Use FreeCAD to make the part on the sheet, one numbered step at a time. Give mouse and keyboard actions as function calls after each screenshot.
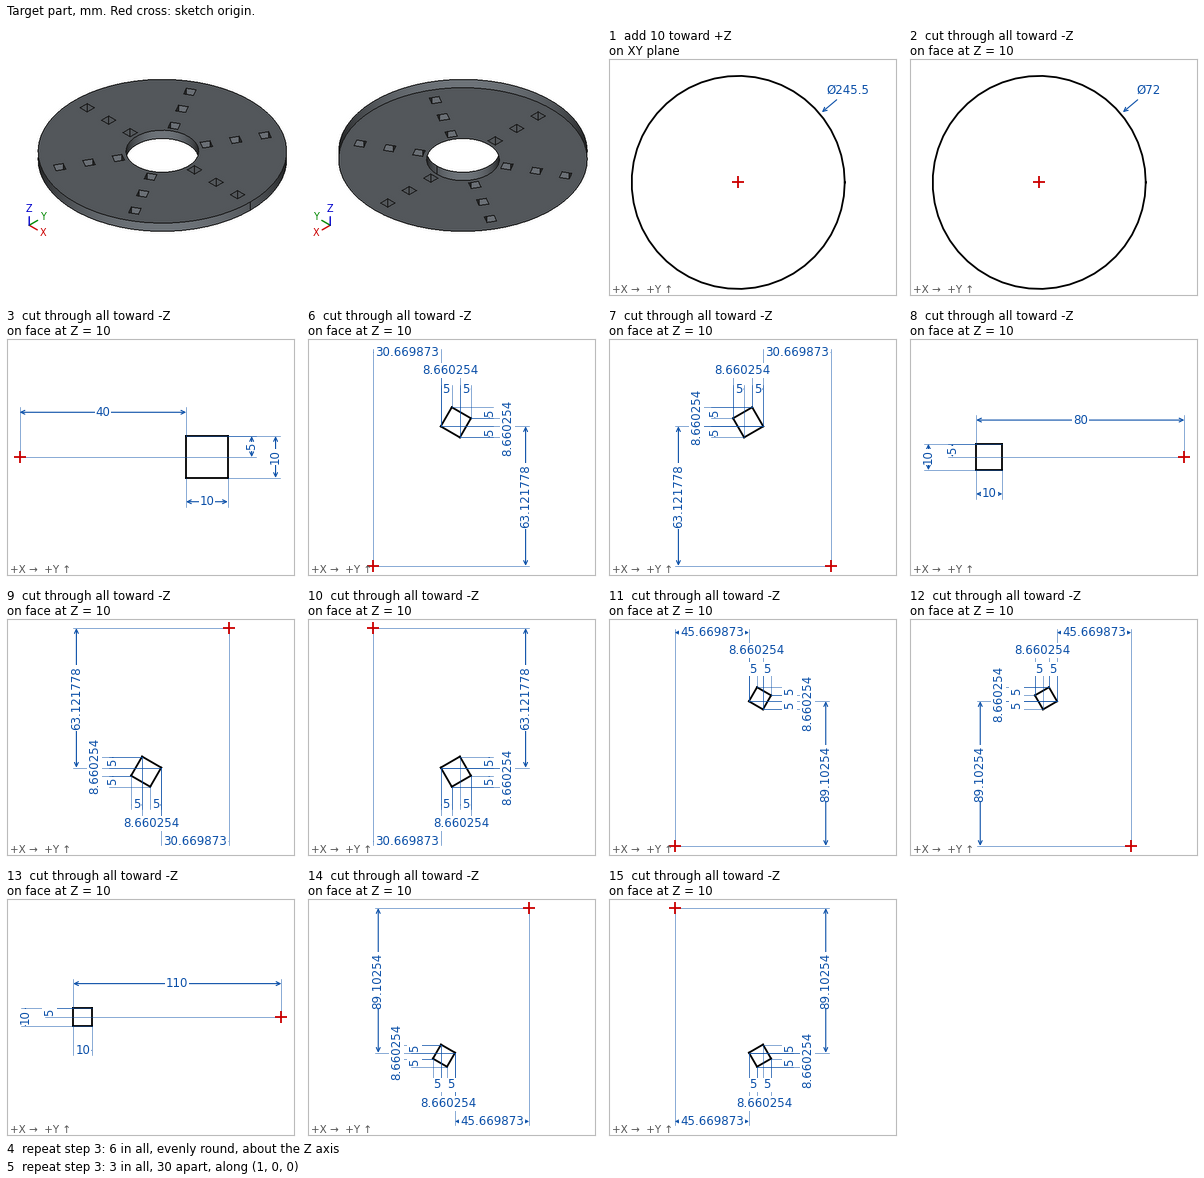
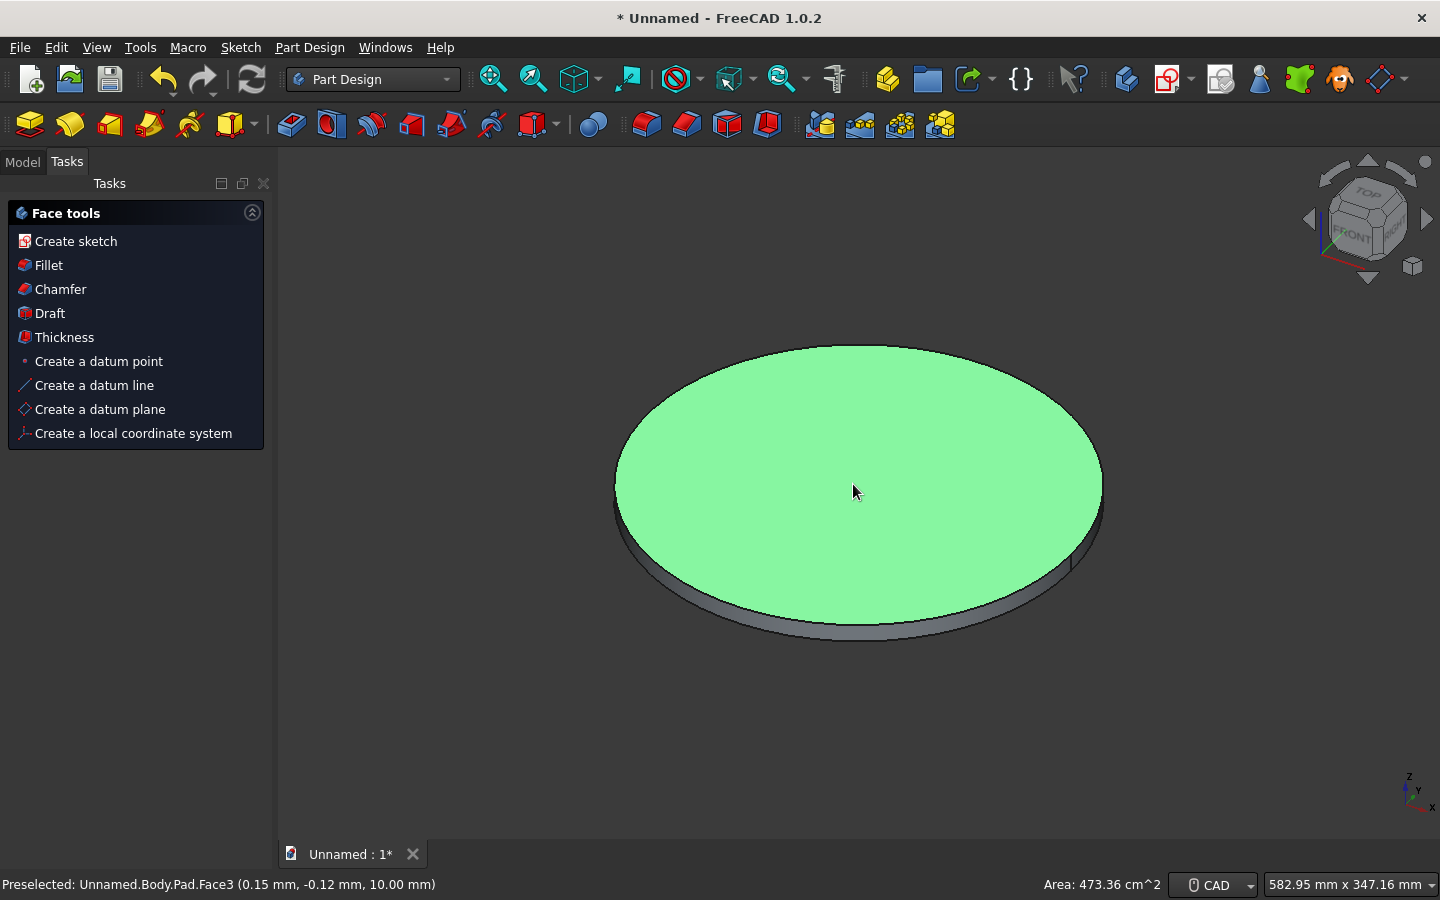
click(1168, 80)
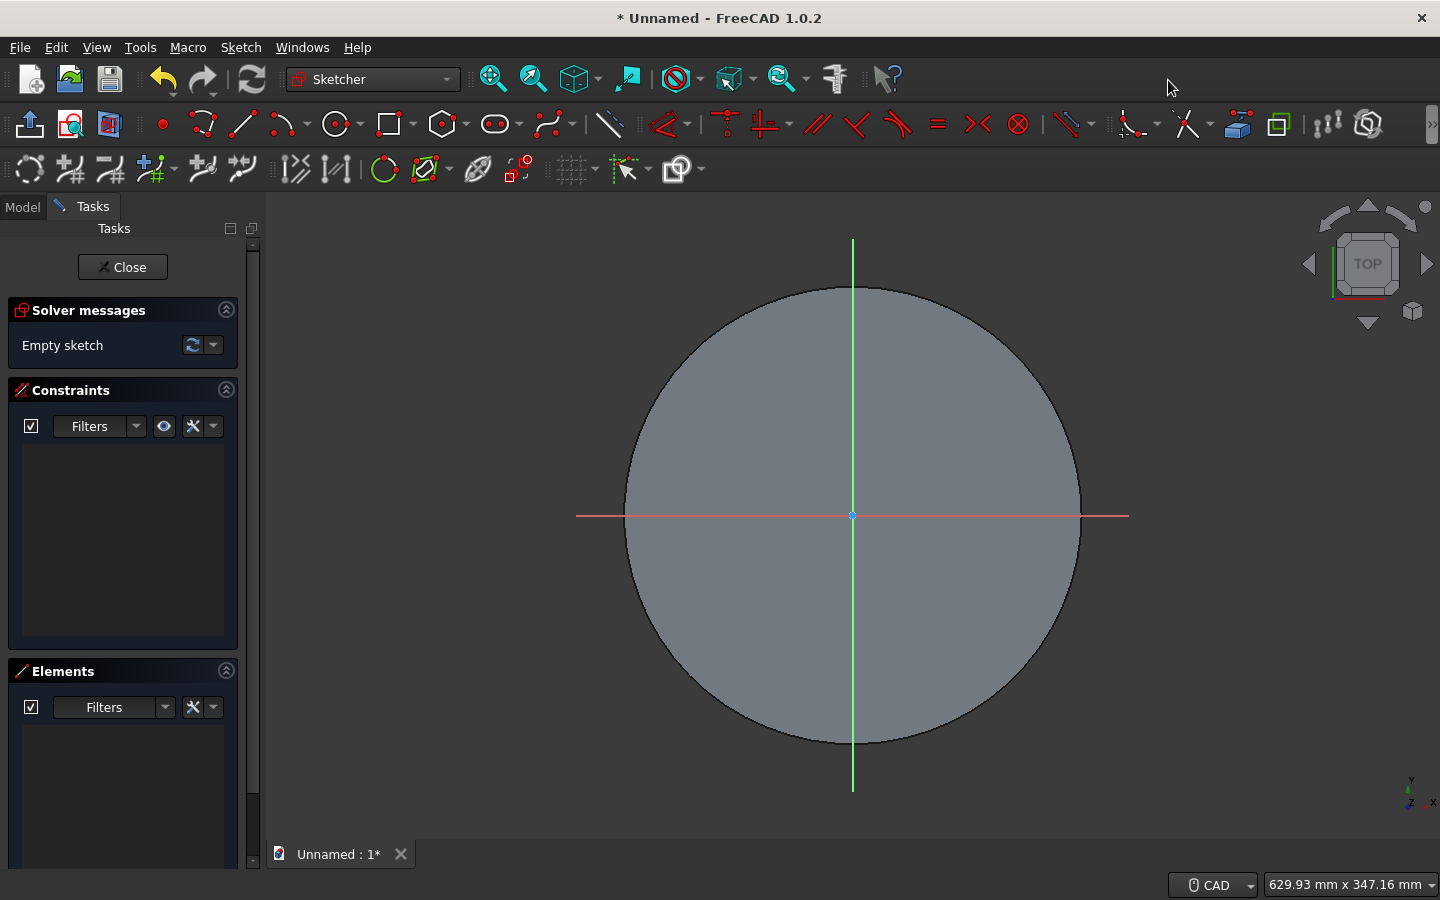
scroll(882, 516, up, 6)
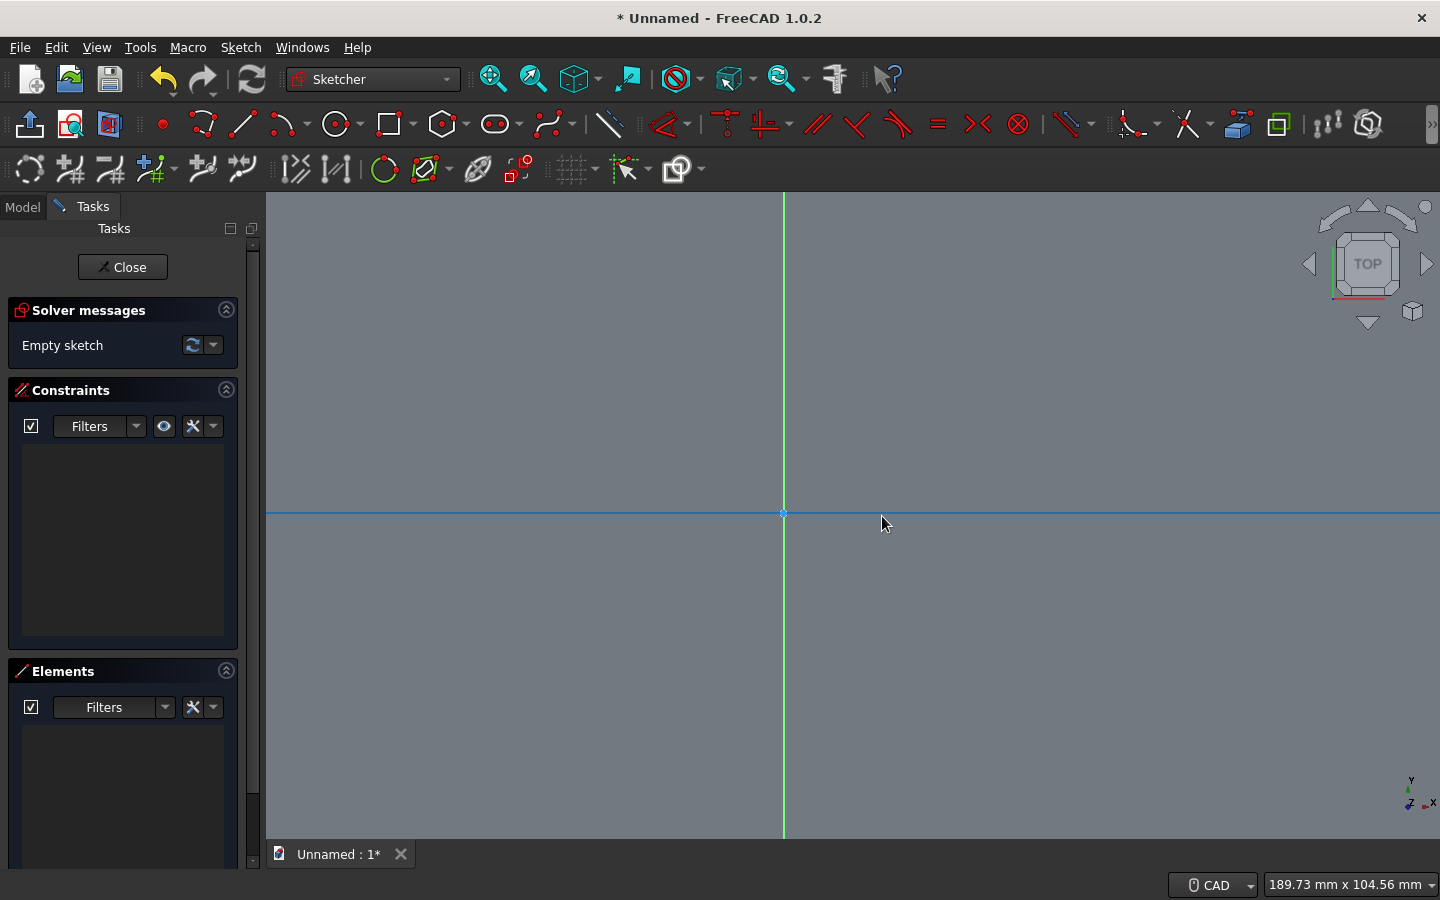
click(336, 124)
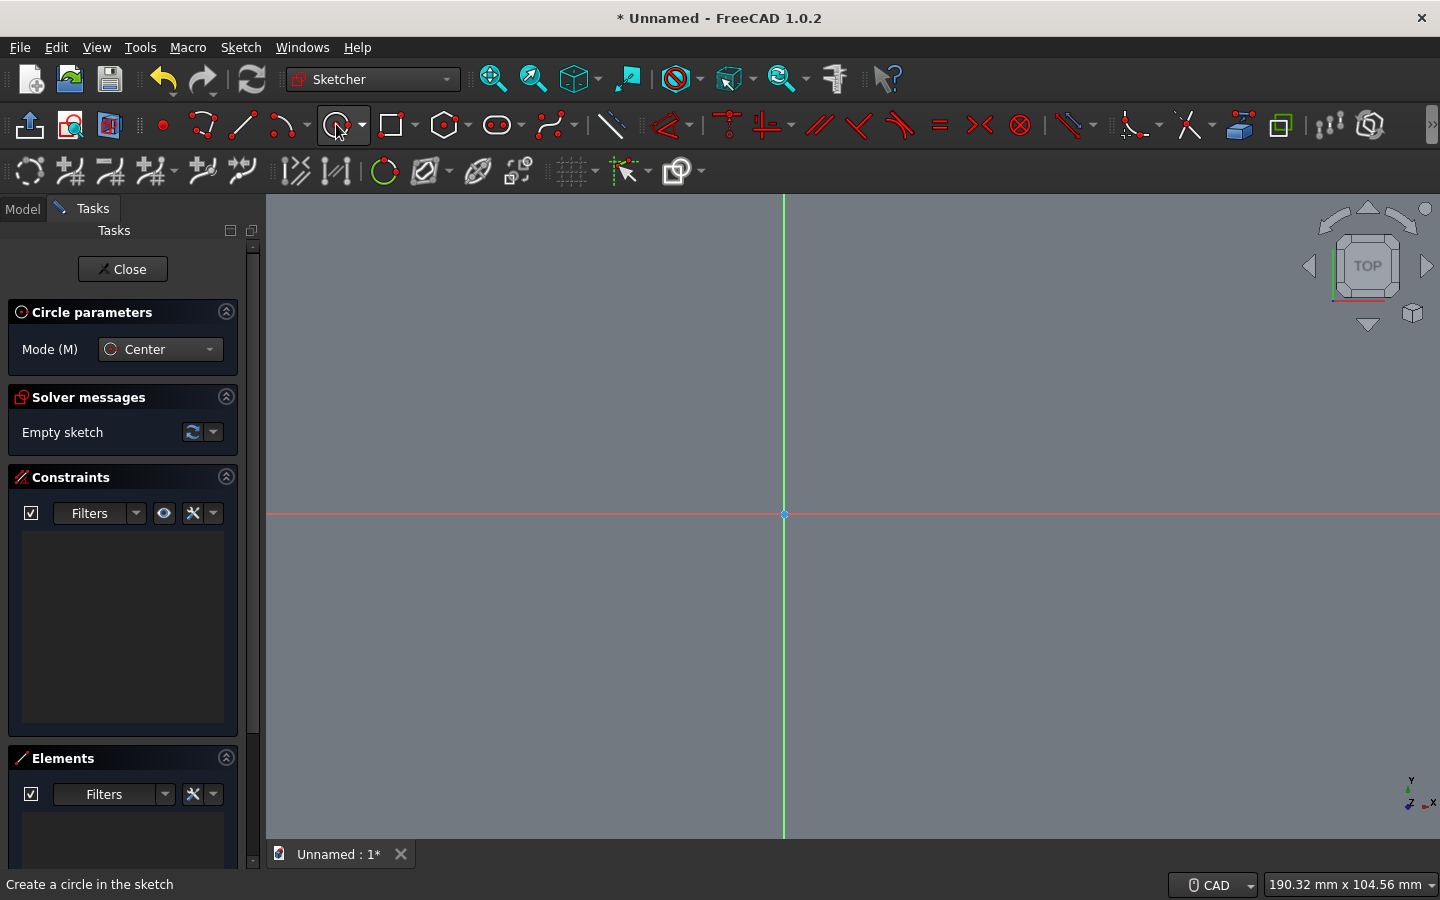
click(784, 514)
move(941, 357)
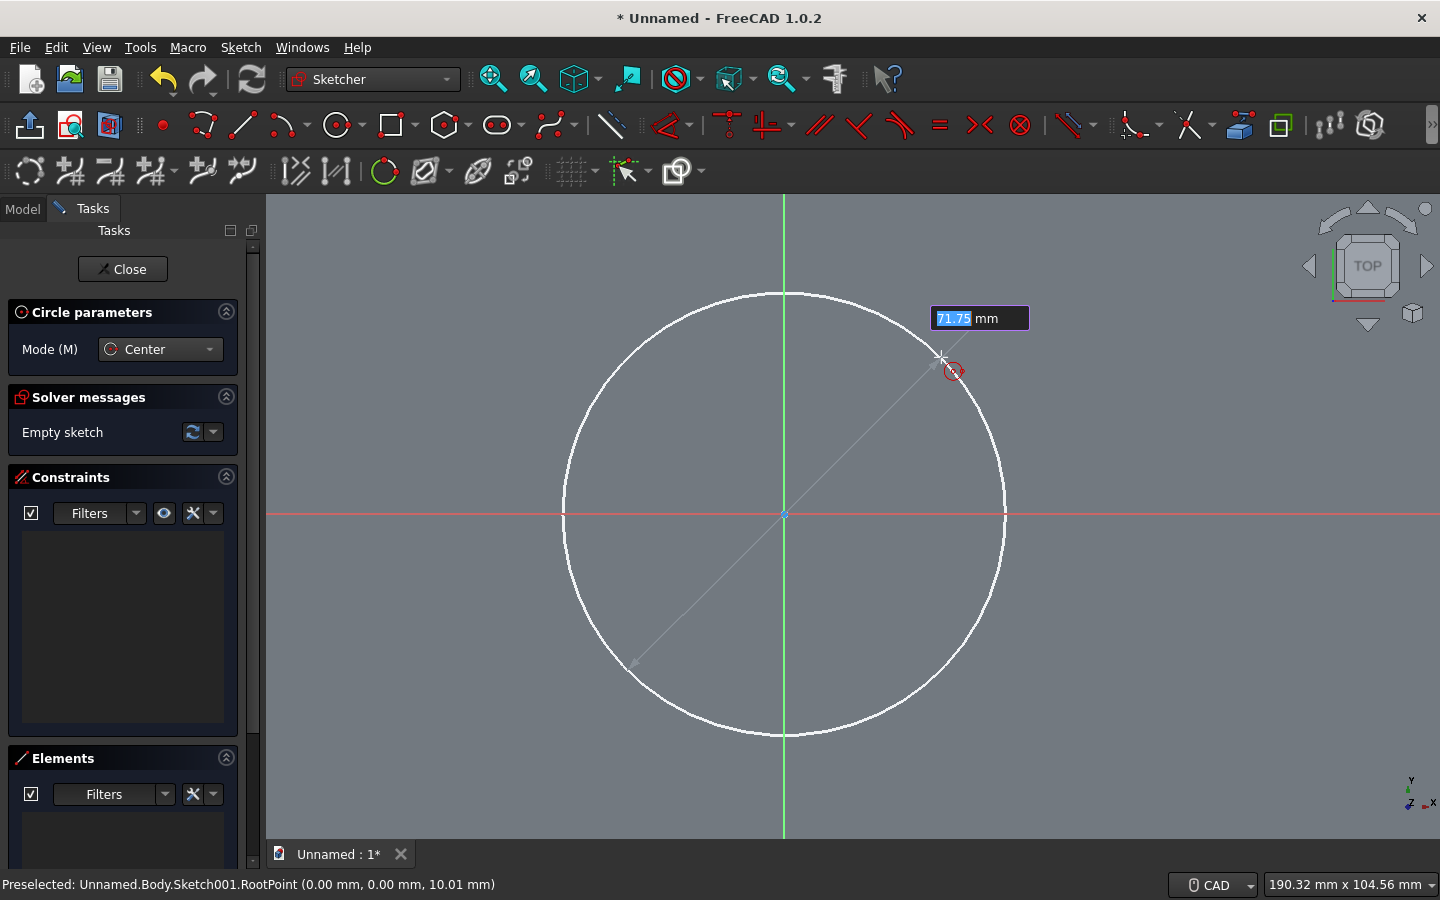
text(72)
key(Return)
key(Escape)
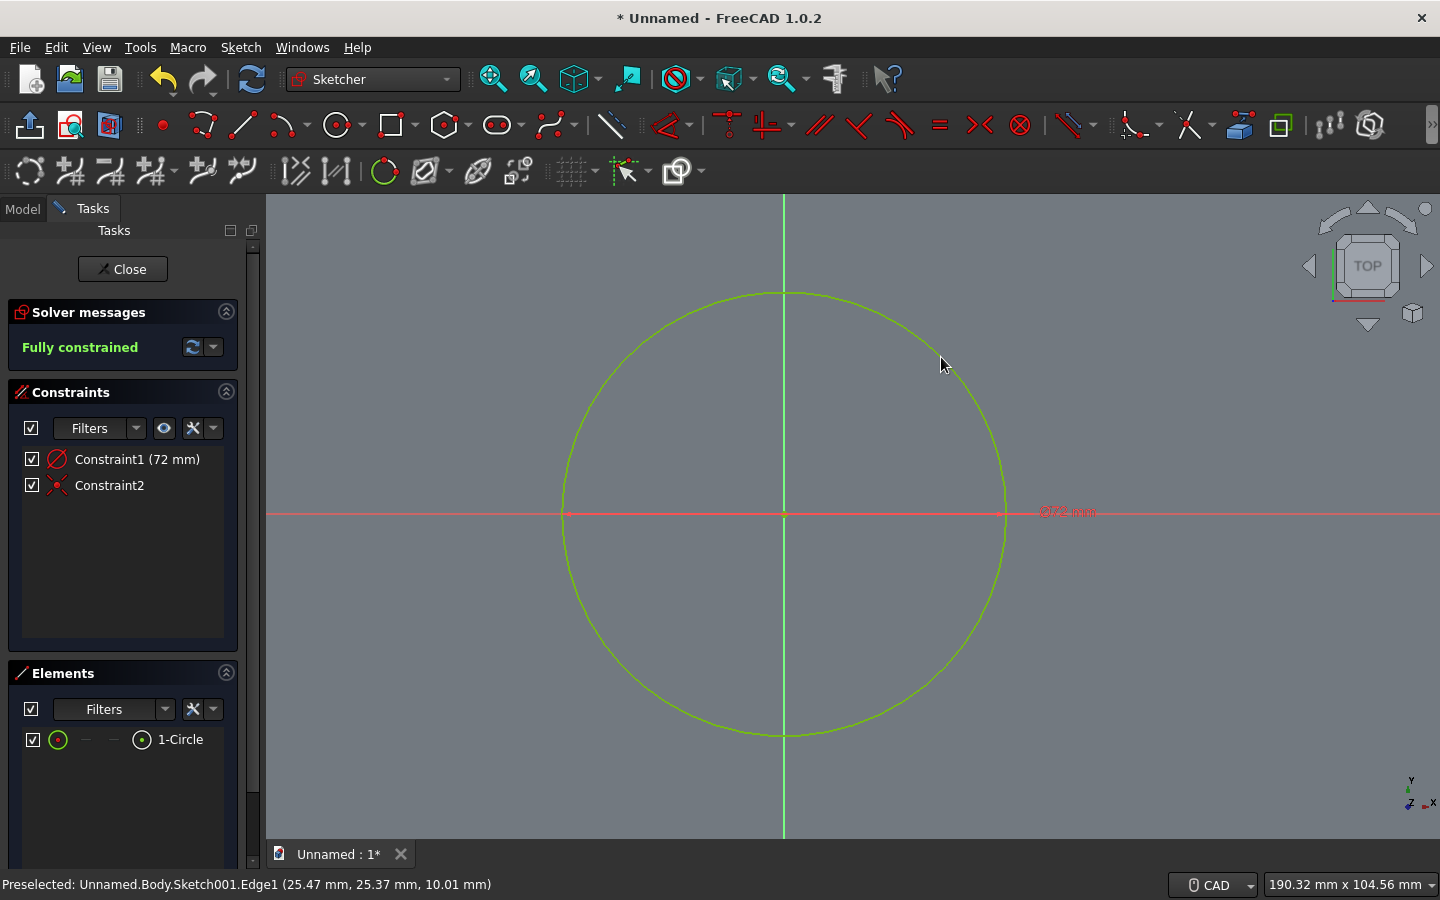
click(123, 269)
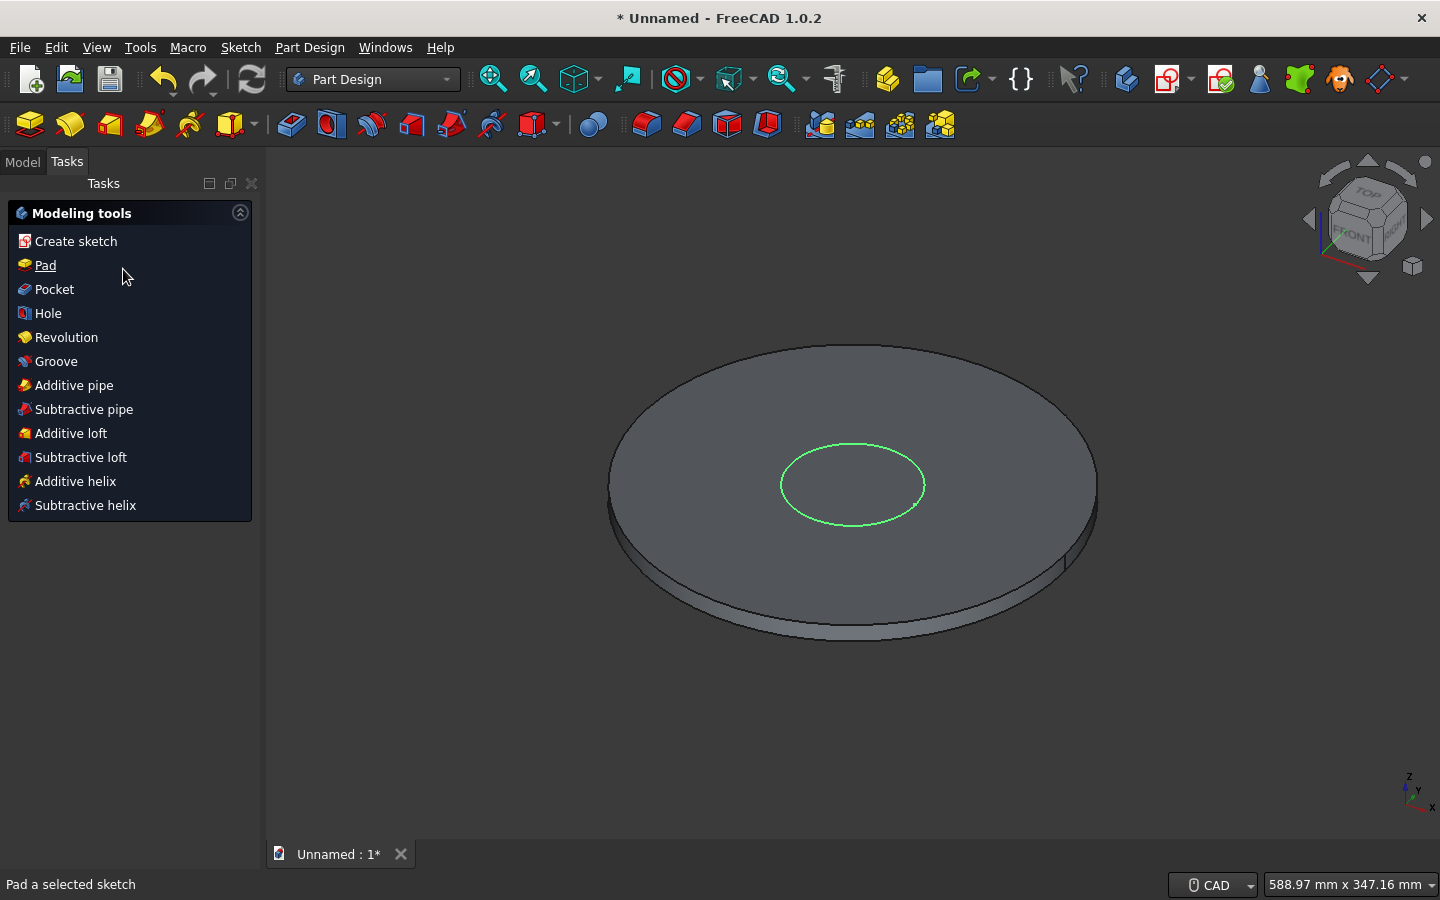
click(292, 124)